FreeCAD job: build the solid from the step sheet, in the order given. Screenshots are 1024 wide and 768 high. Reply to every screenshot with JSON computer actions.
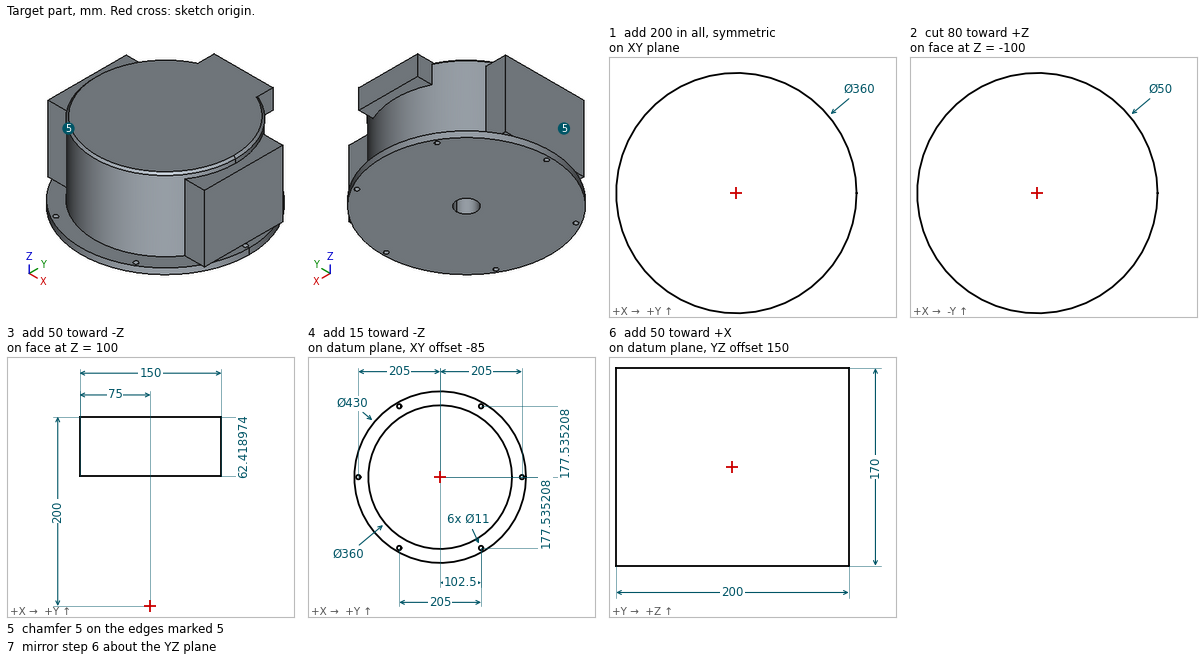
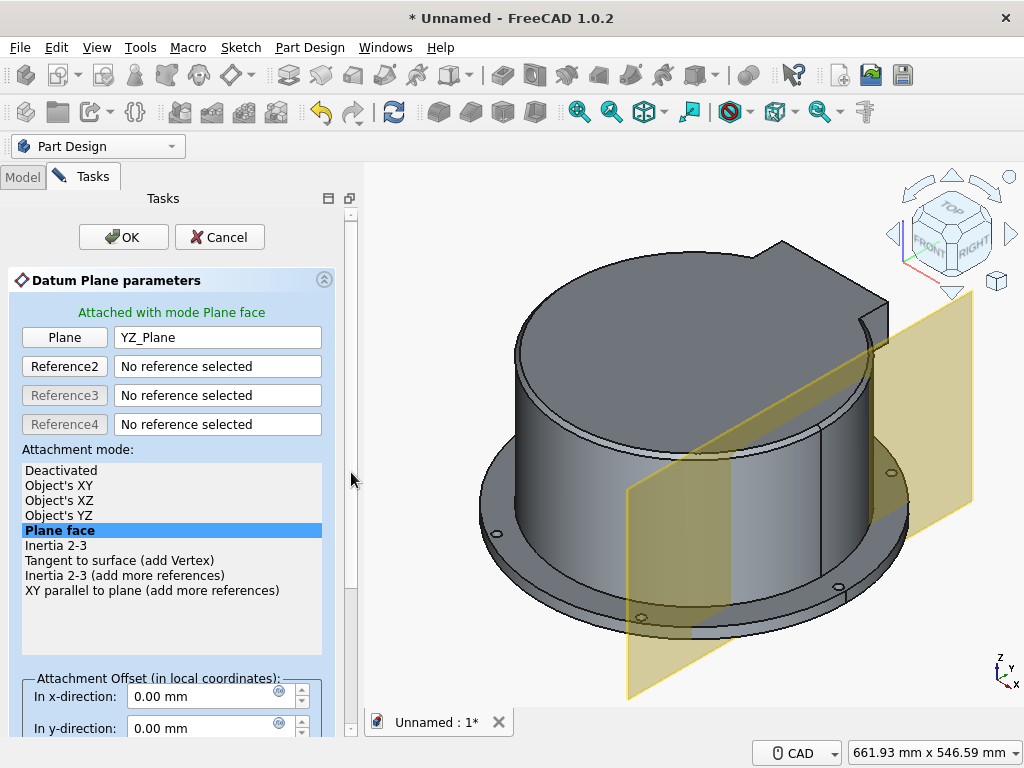
{"action": "left_click", "coordinate": [124, 237]}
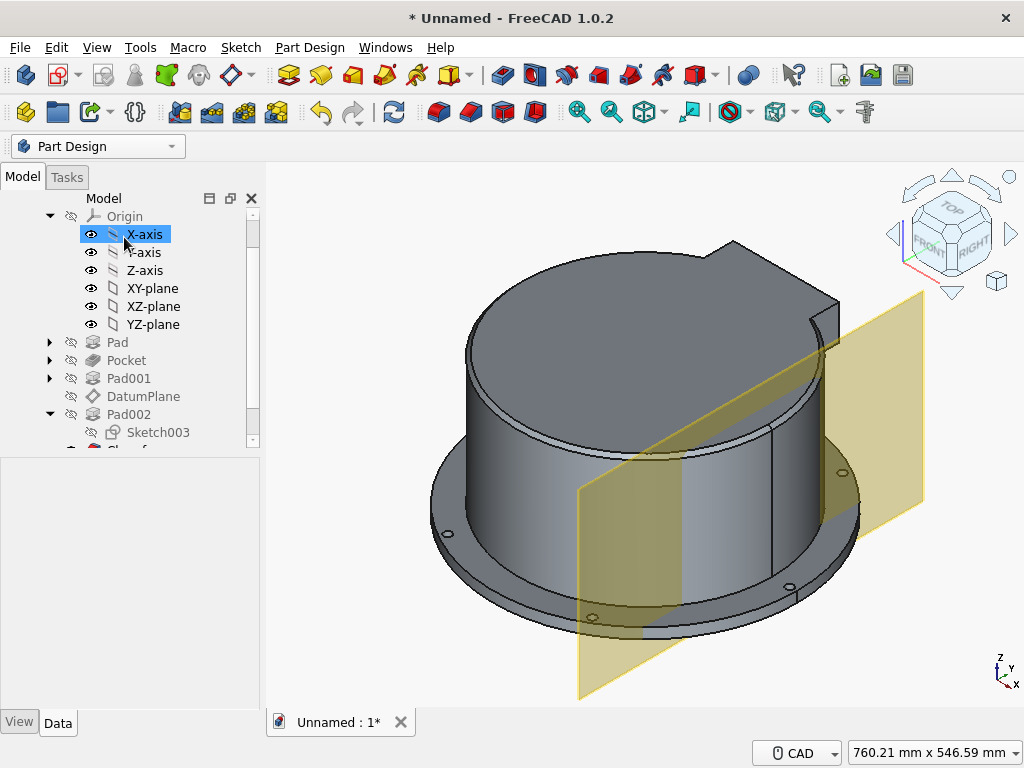
{"action": "scroll", "coordinate": [140, 320], "scroll_direction": "down", "scroll_amount": 3}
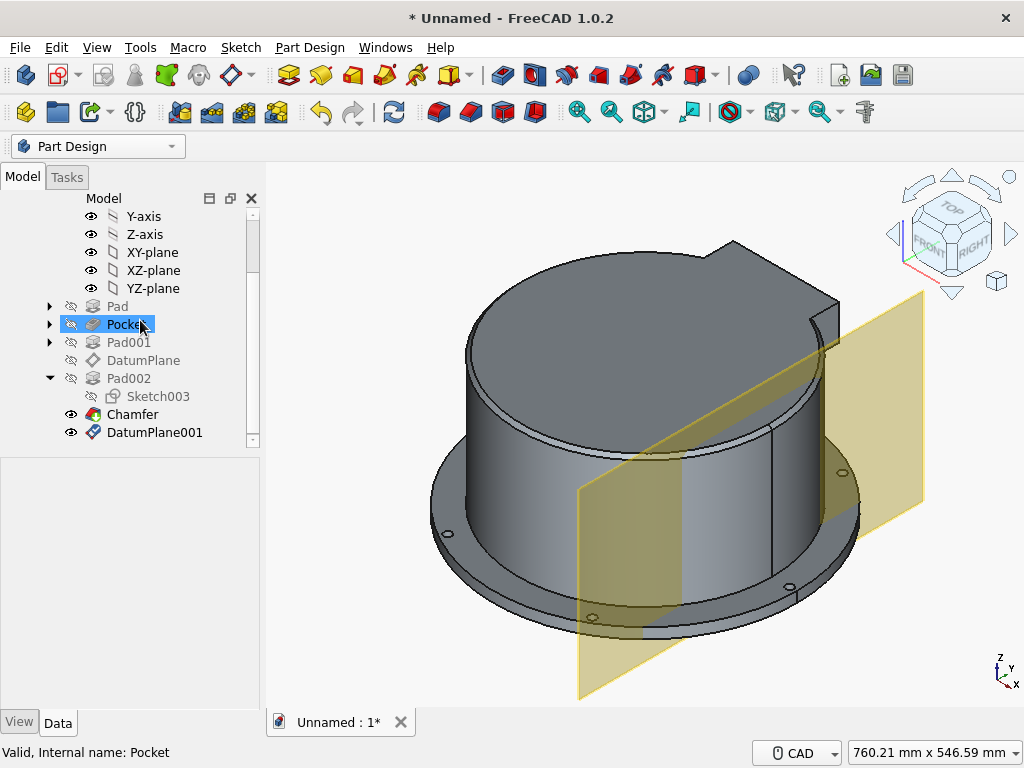
{"action": "left_click", "coordinate": [116, 432]}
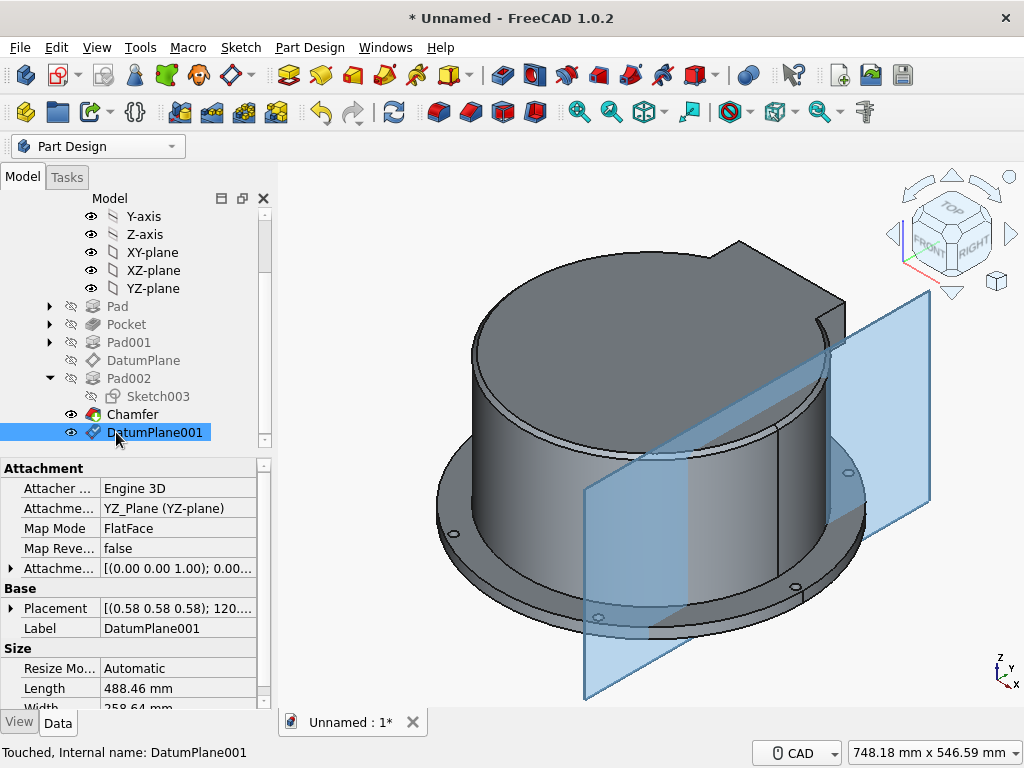
{"action": "left_click", "coordinate": [58, 76]}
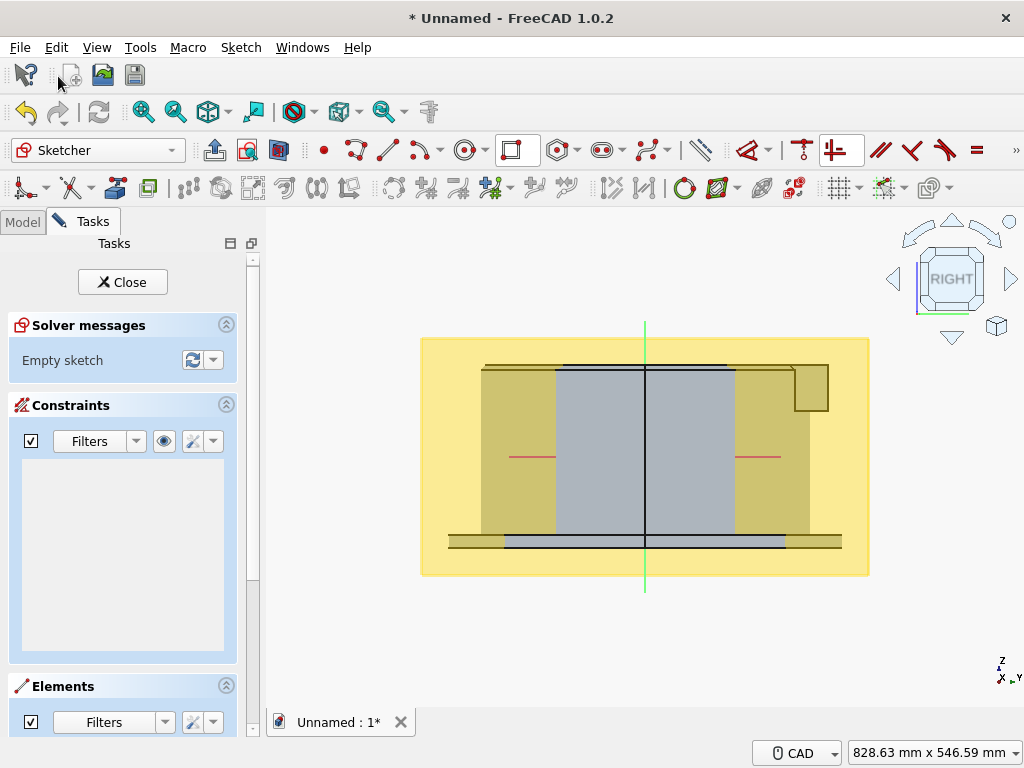
{"action": "key", "text": "q s"}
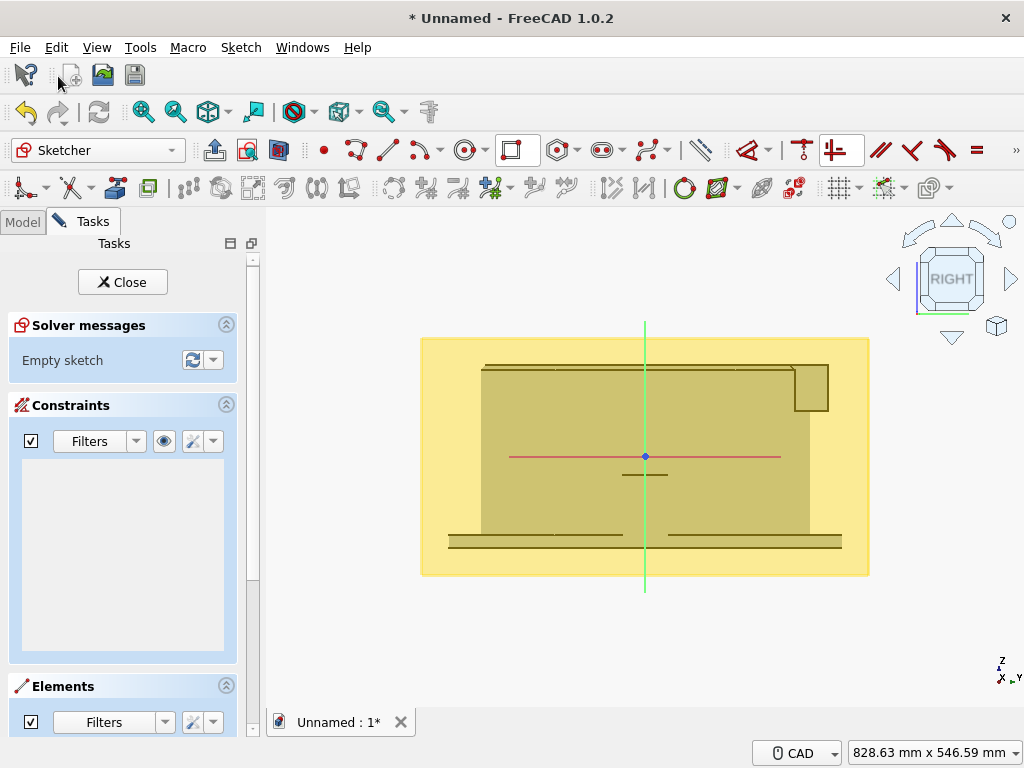
{"action": "scroll", "coordinate": [701, 457], "scroll_direction": "up", "scroll_amount": 4}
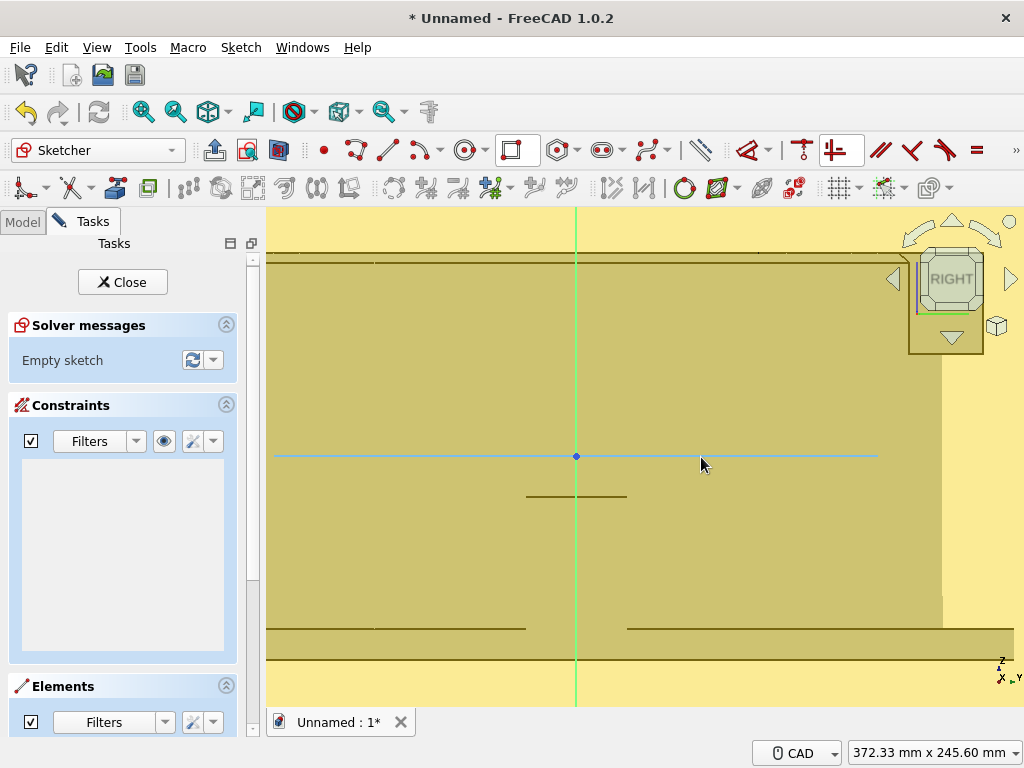
{"action": "key", "text": "g v"}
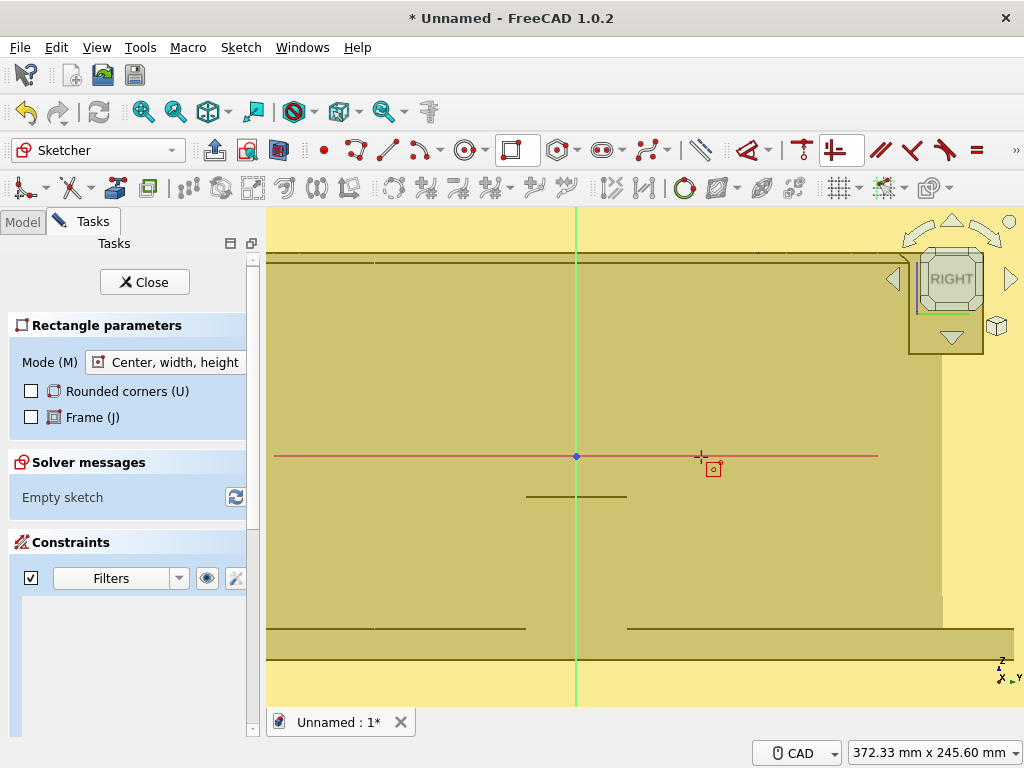
{"action": "left_click", "coordinate": [576, 456]}
{"action": "mouse_move", "coordinate": [780, 283]}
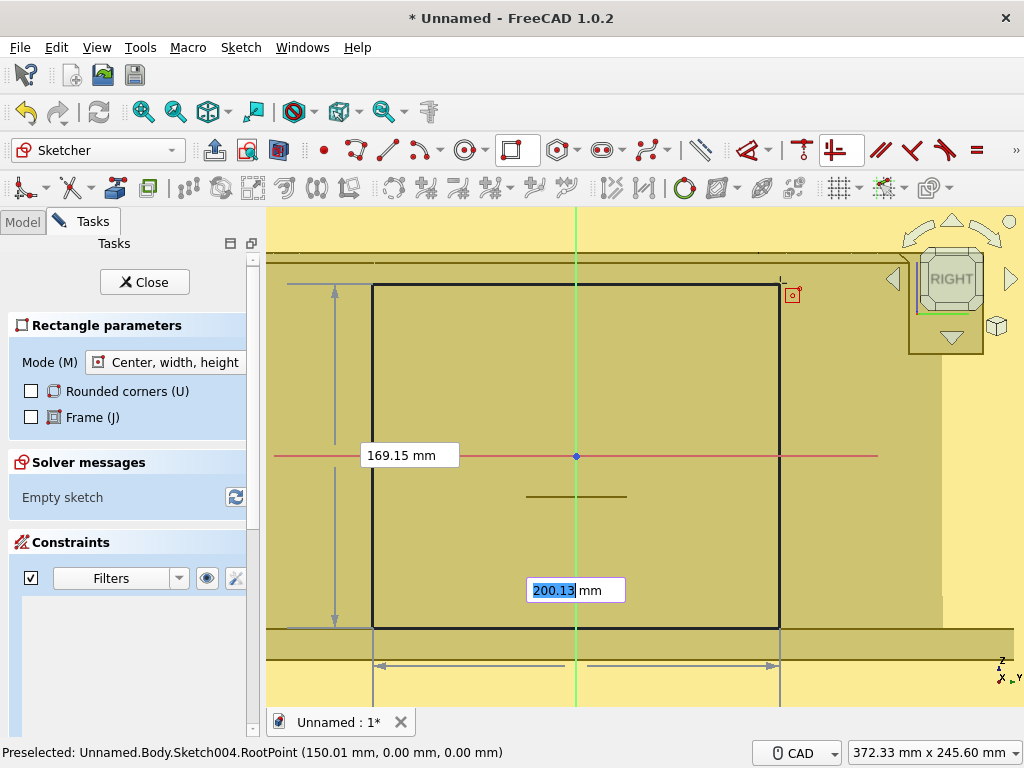
{"action": "type", "text": "200"}
{"action": "key", "text": "Tab"}
{"action": "type", "text": "170"}
{"action": "key", "text": "Return"}
{"action": "key", "text": "Escape"}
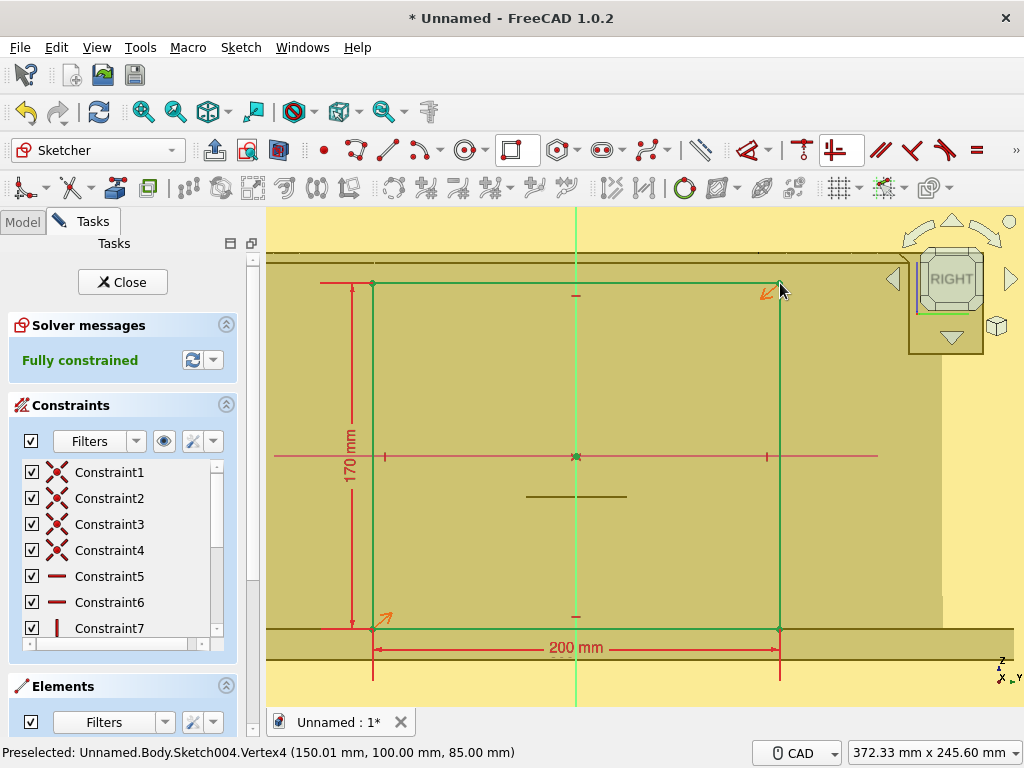
{"action": "left_click", "coordinate": [123, 282]}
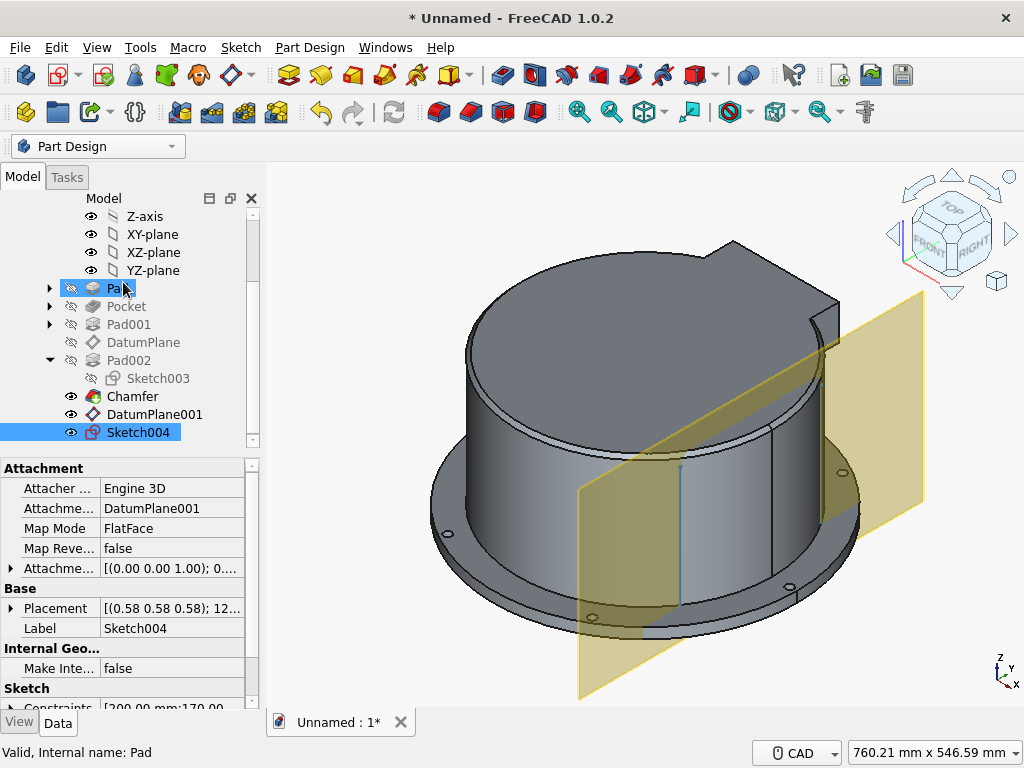
{"action": "left_click", "coordinate": [290, 76]}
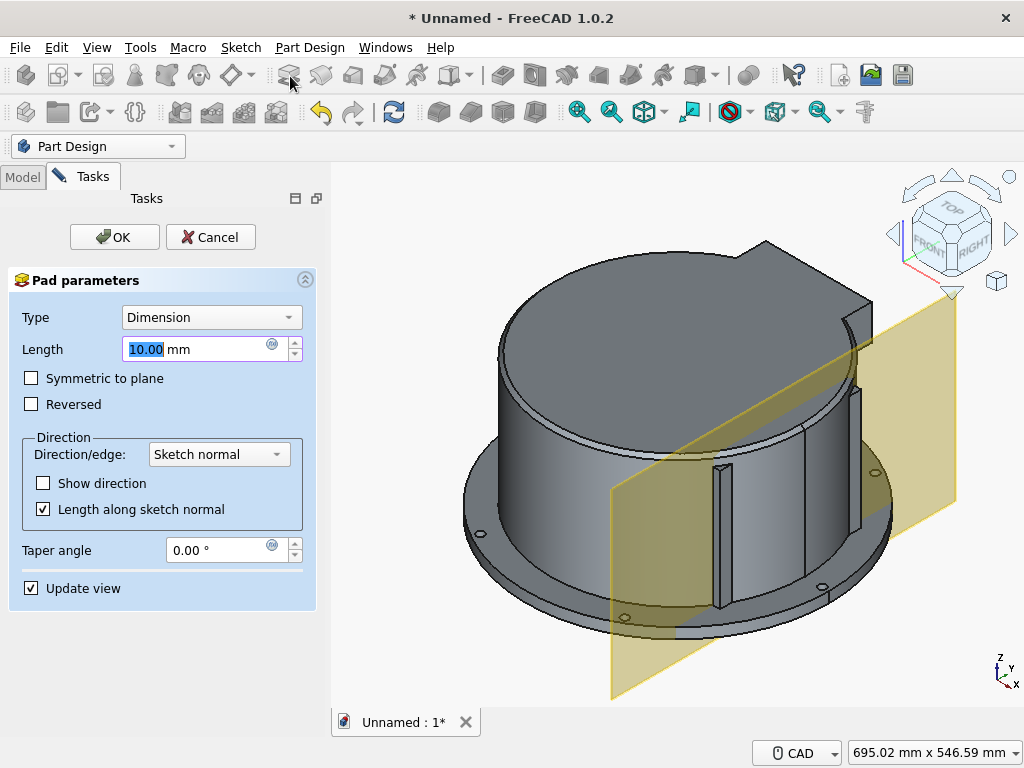
{"action": "type", "text": "50"}
{"action": "key", "text": "Tab"}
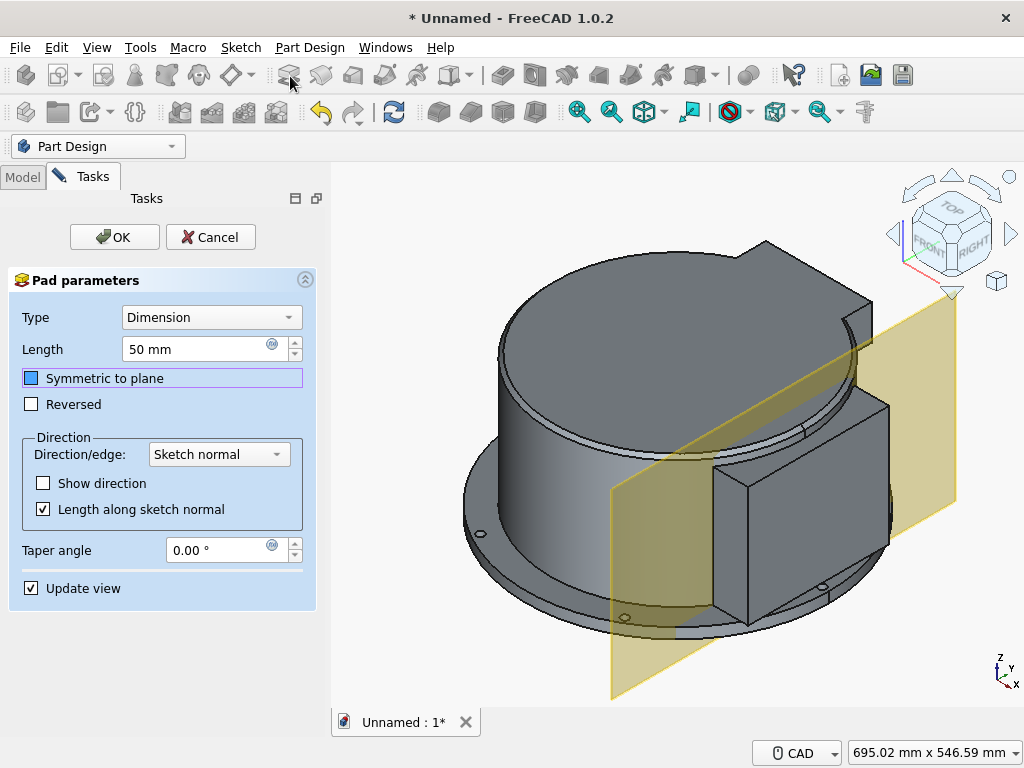
{"action": "left_click", "coordinate": [115, 237]}